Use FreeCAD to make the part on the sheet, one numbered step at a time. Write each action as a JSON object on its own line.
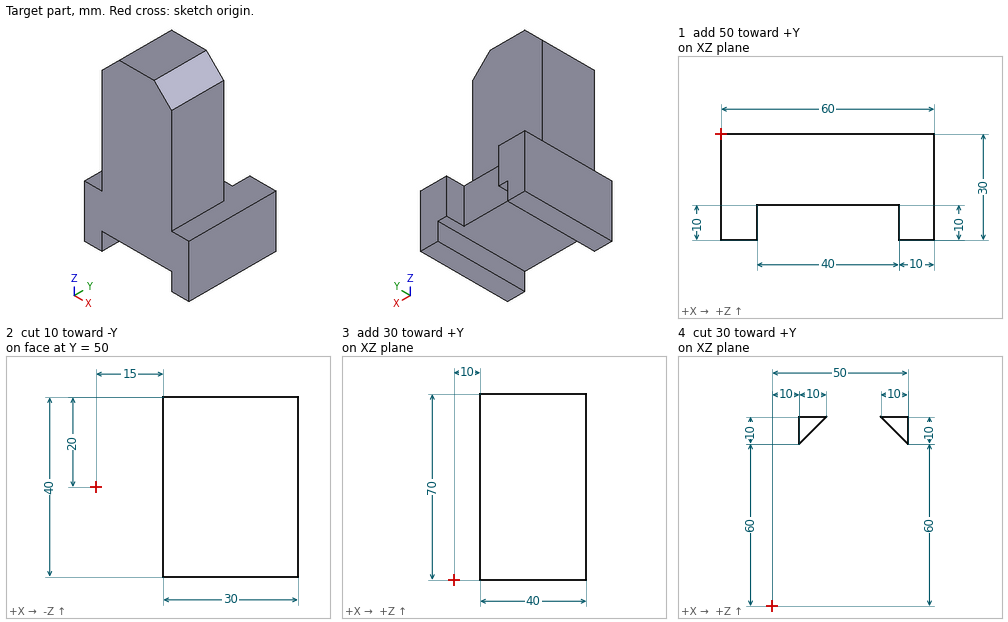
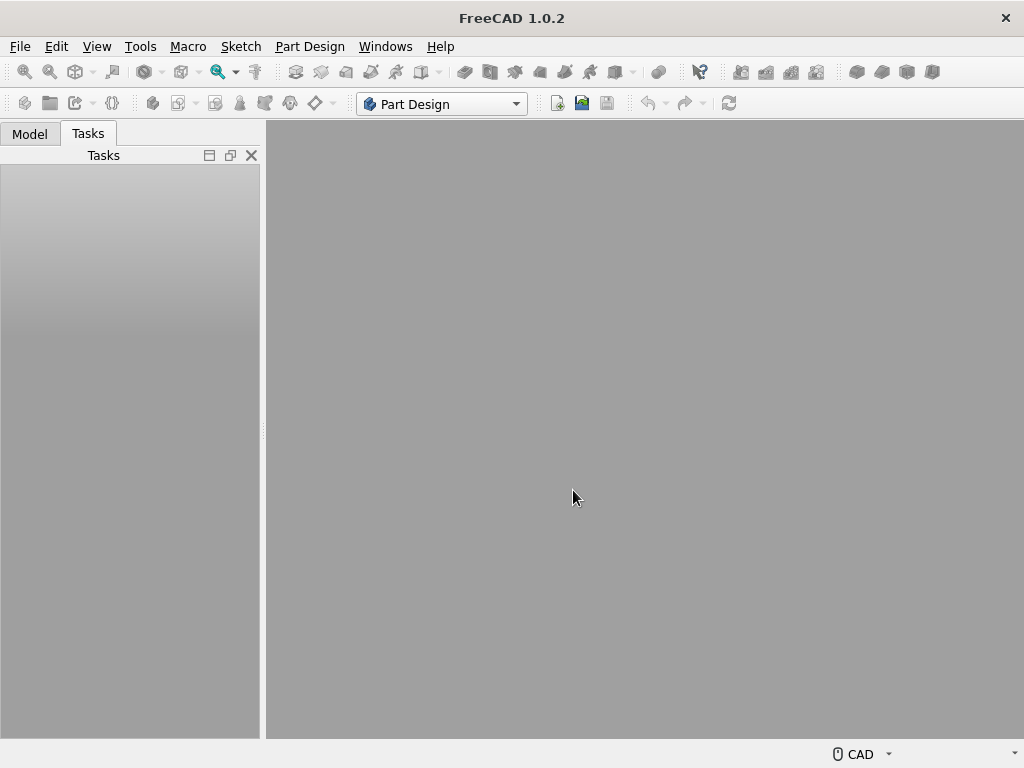
{"action": "left_click", "coordinate": [557, 104]}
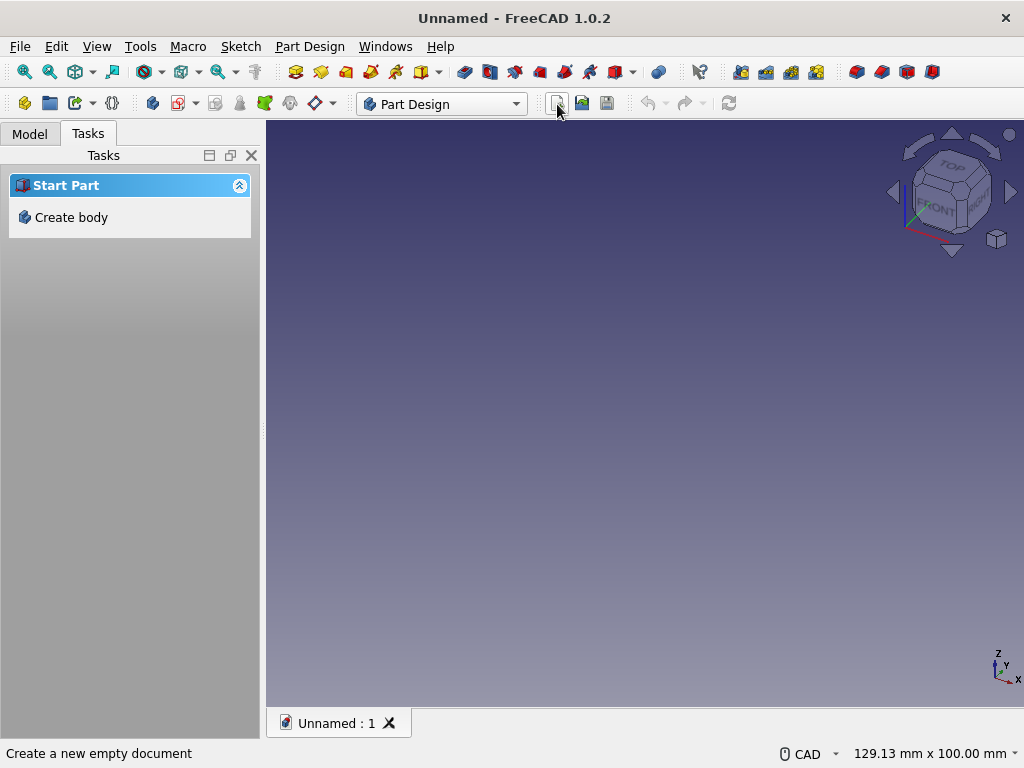
{"action": "left_click", "coordinate": [178, 104]}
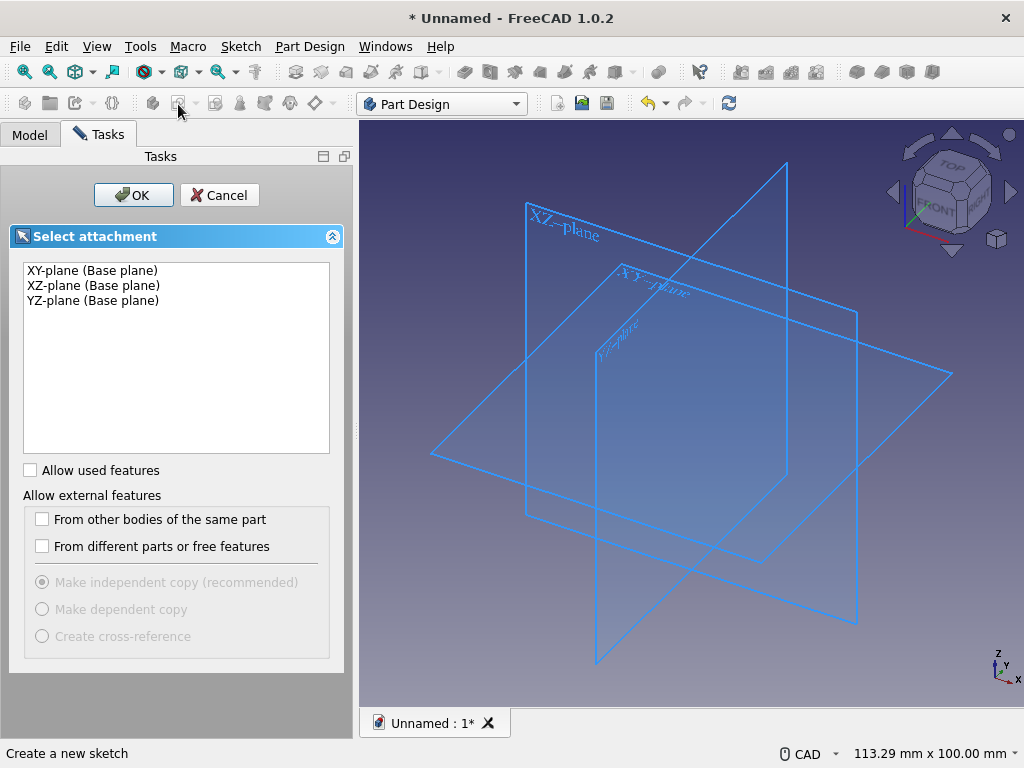
{"action": "left_click", "coordinate": [84, 286]}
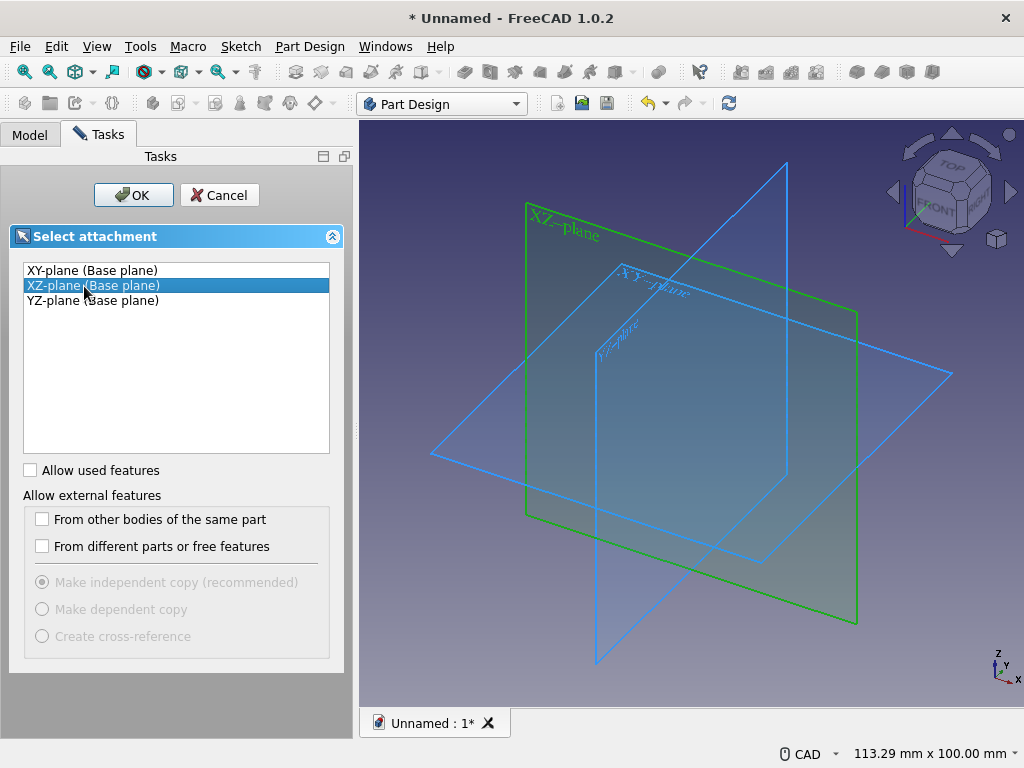
{"action": "left_click", "coordinate": [134, 195]}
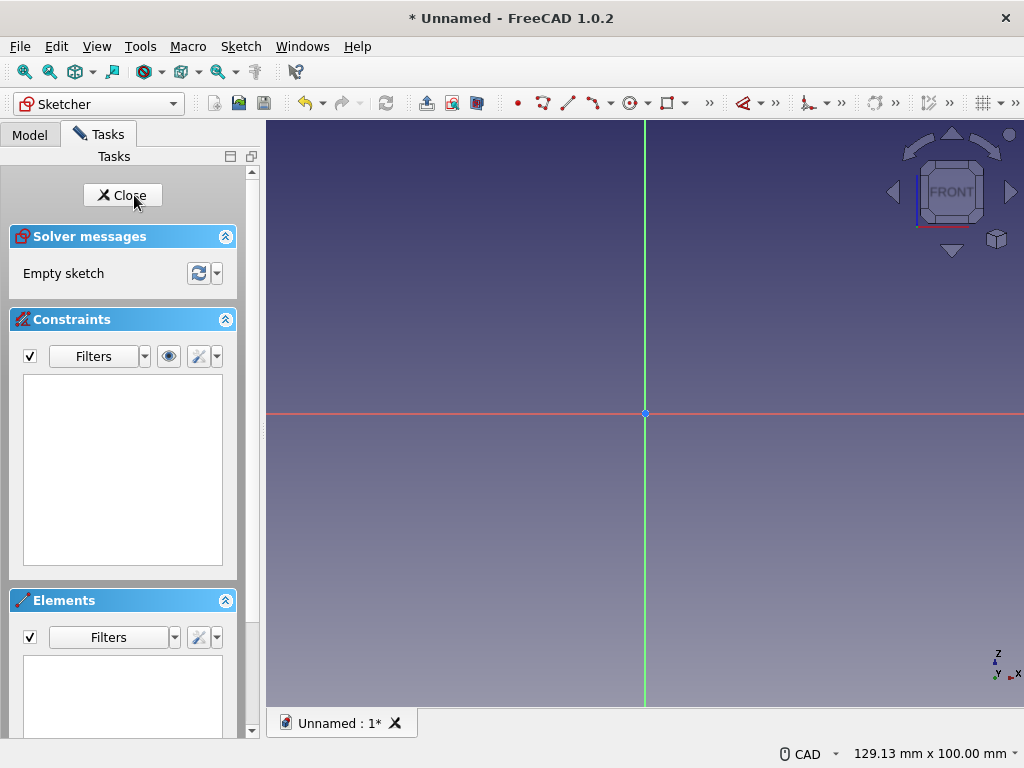
{"action": "scroll", "coordinate": [294, 234], "scroll_direction": "down", "scroll_amount": 2}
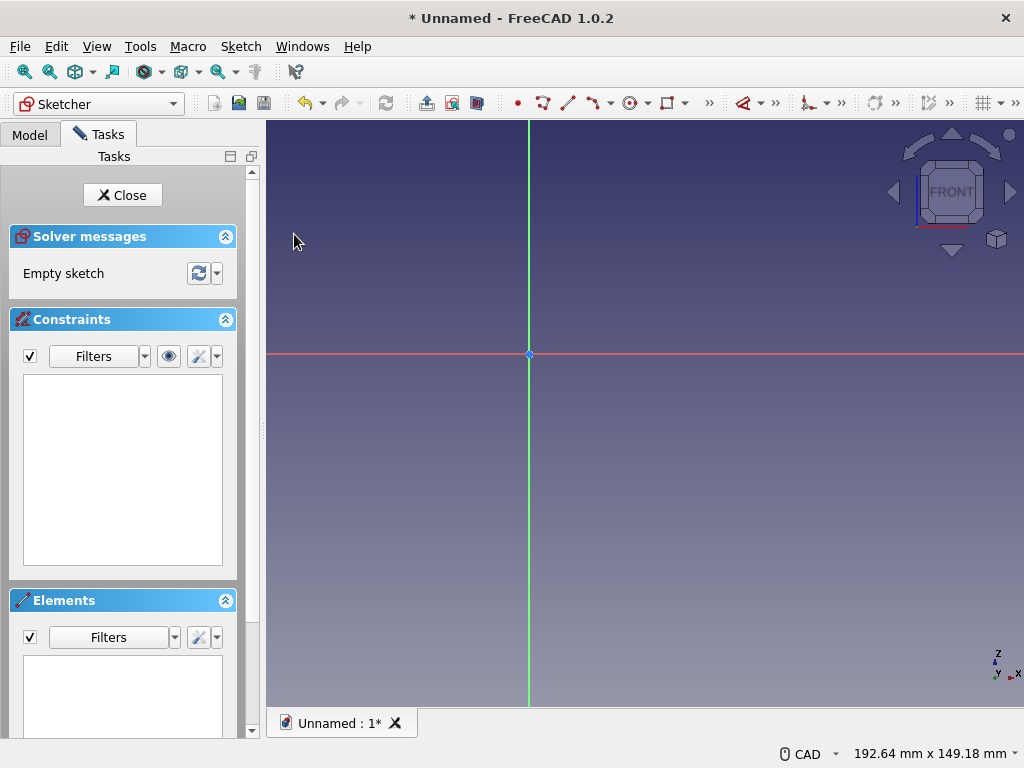
{"action": "scroll", "coordinate": [734, 413], "scroll_direction": "up", "scroll_amount": 3}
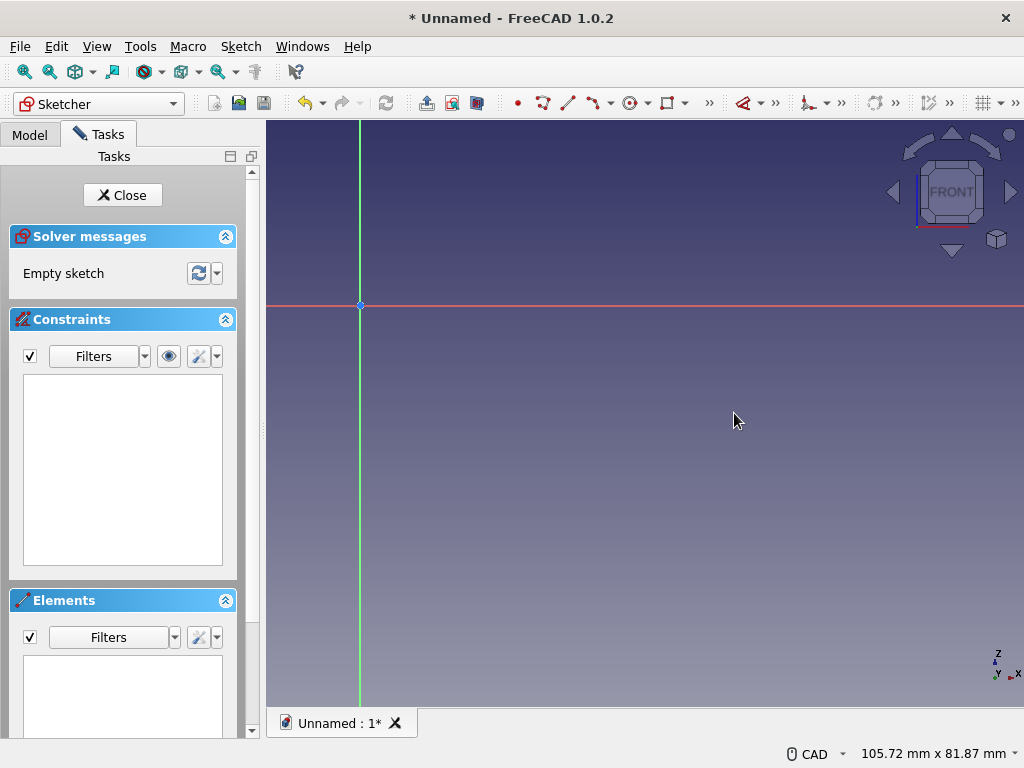
{"action": "left_click", "coordinate": [543, 104]}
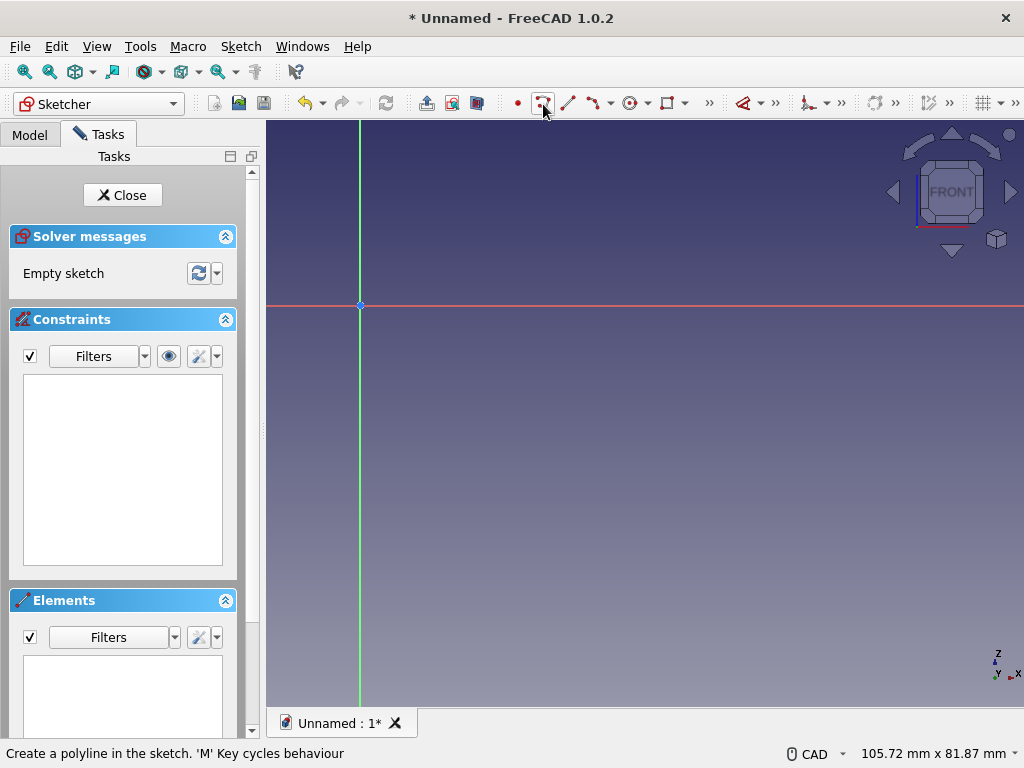
{"action": "left_click", "coordinate": [360, 306]}
{"action": "left_click", "coordinate": [791, 315]}
{"action": "left_click", "coordinate": [791, 521]}
{"action": "left_click", "coordinate": [719, 521]}
{"action": "left_click", "coordinate": [719, 449]}
{"action": "left_click", "coordinate": [432, 449]}
{"action": "left_click", "coordinate": [432, 521]}
{"action": "left_click", "coordinate": [369, 521]}
{"action": "left_click", "coordinate": [360, 306]}
{"action": "key", "text": "Escape"}
{"action": "key", "text": "Escape"}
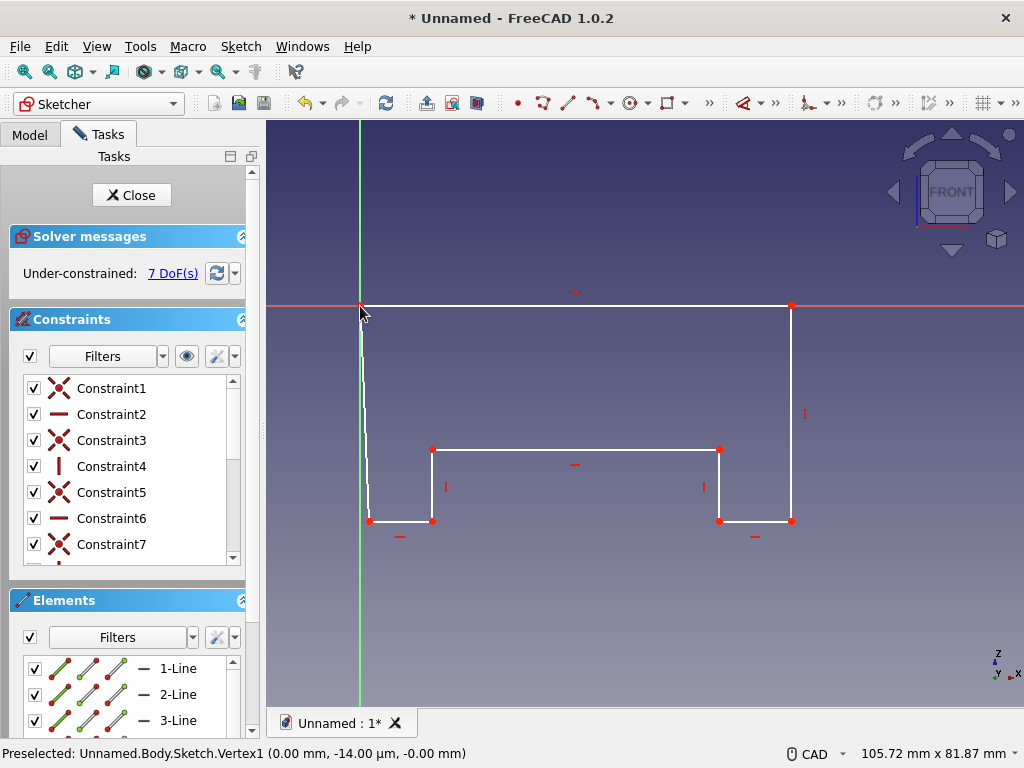
{"action": "left_click", "coordinate": [363, 371]}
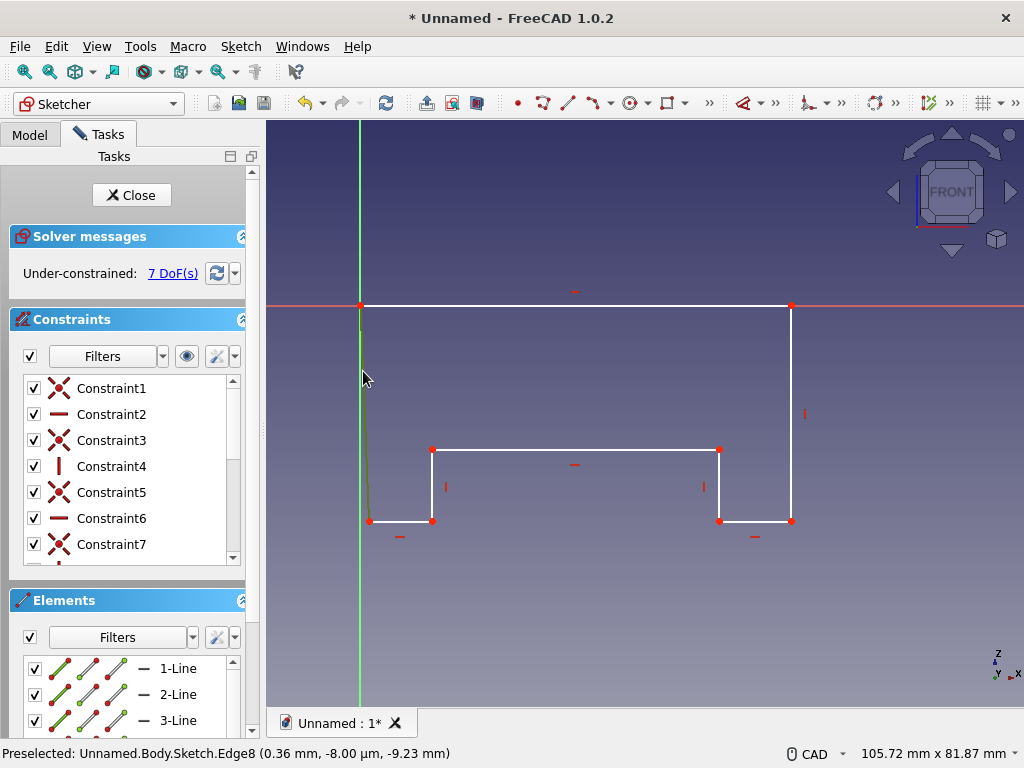
{"action": "key", "text": "v"}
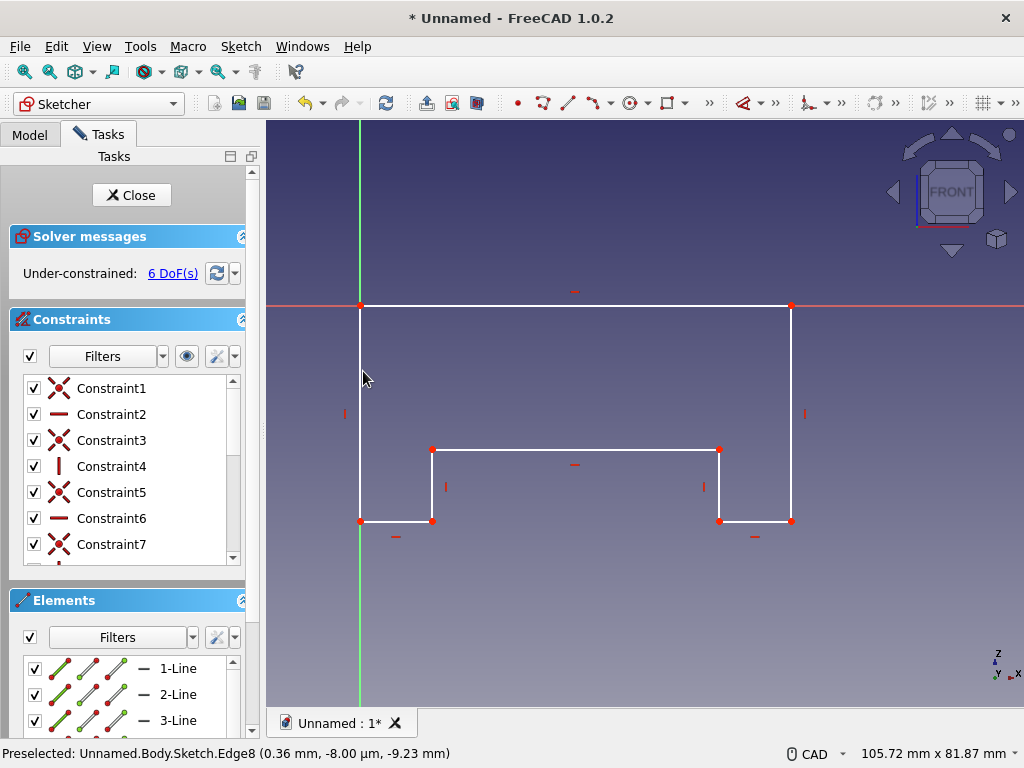
{"action": "left_click", "coordinate": [742, 104]}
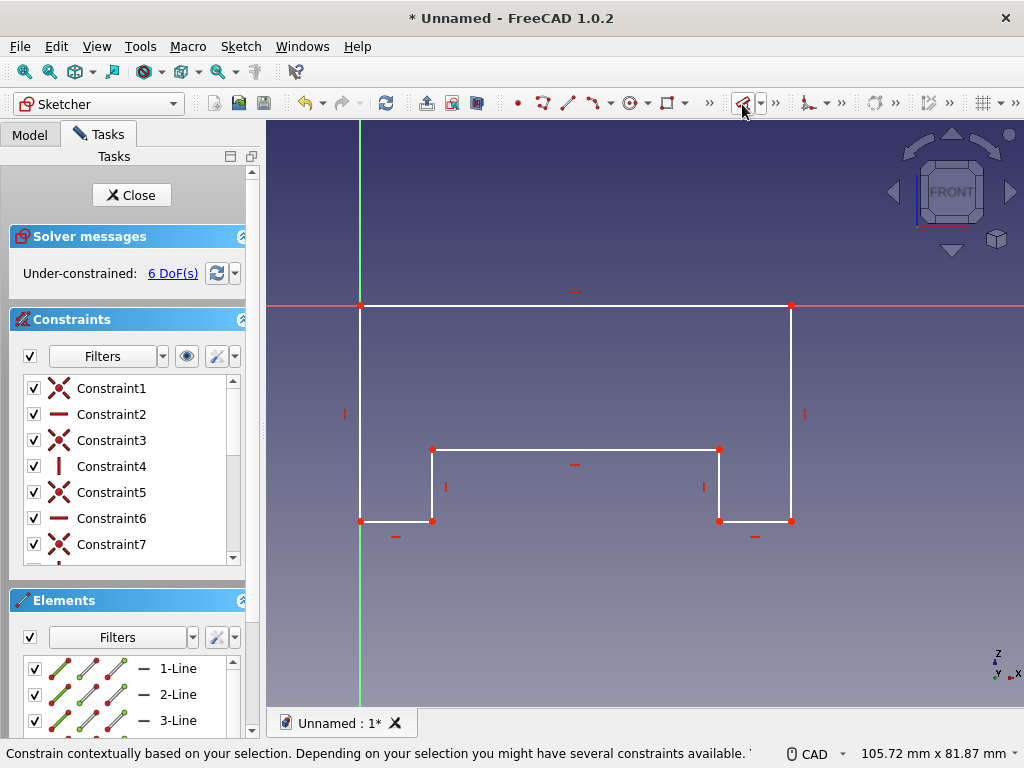
{"action": "left_click", "coordinate": [490, 306]}
{"action": "left_click", "coordinate": [576, 272]}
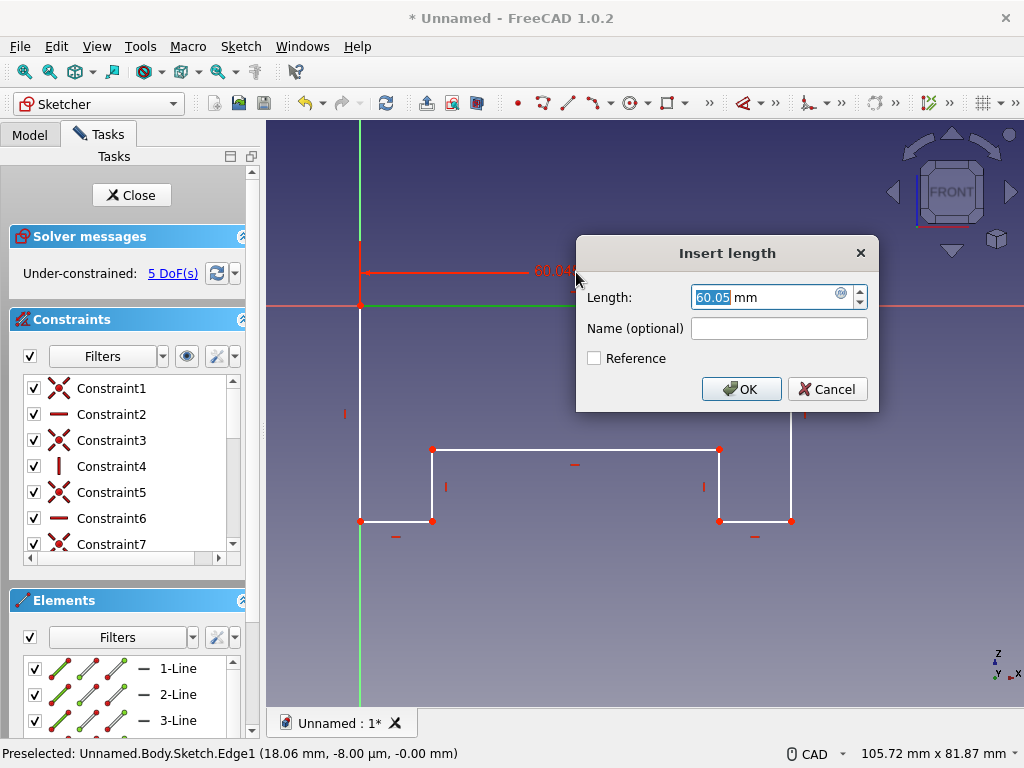
{"action": "type", "text": "60"}
{"action": "key", "text": "Return"}